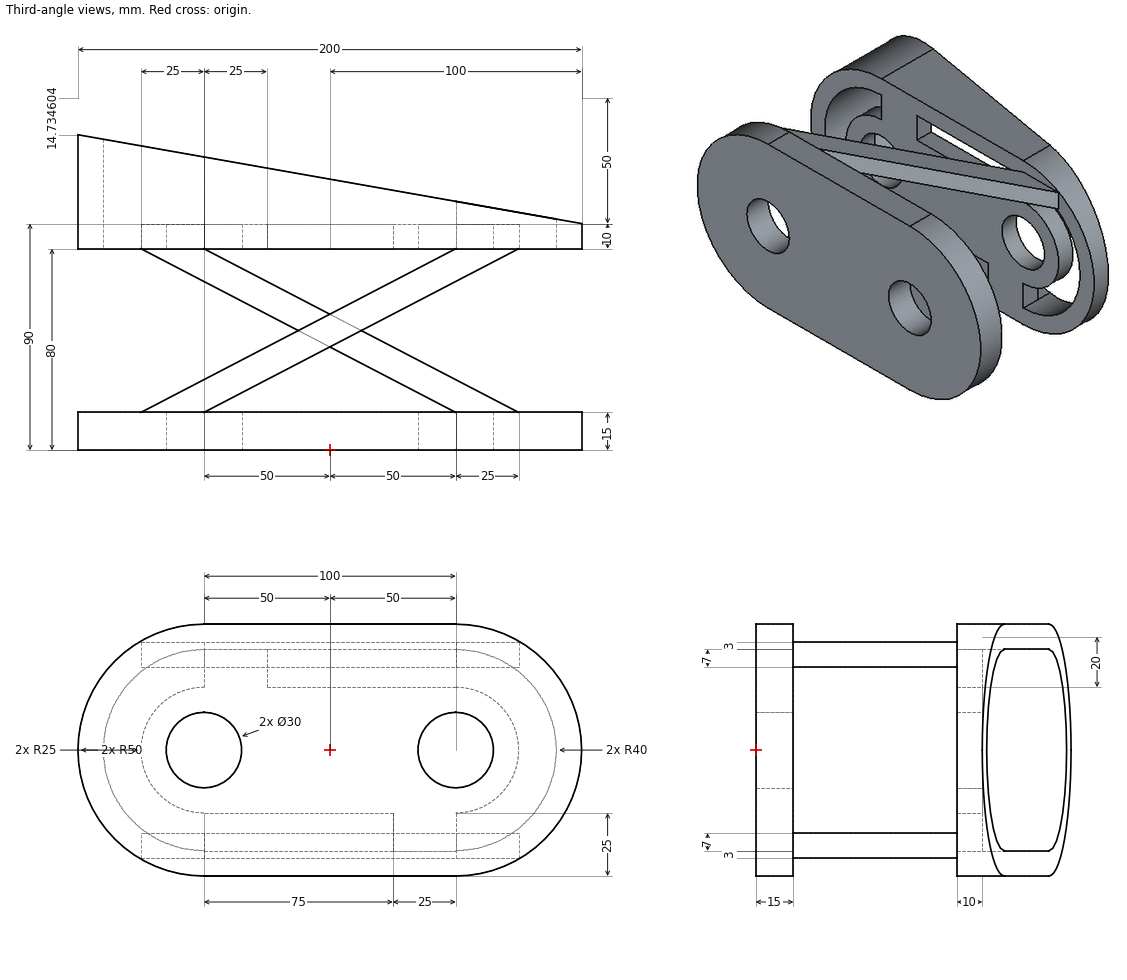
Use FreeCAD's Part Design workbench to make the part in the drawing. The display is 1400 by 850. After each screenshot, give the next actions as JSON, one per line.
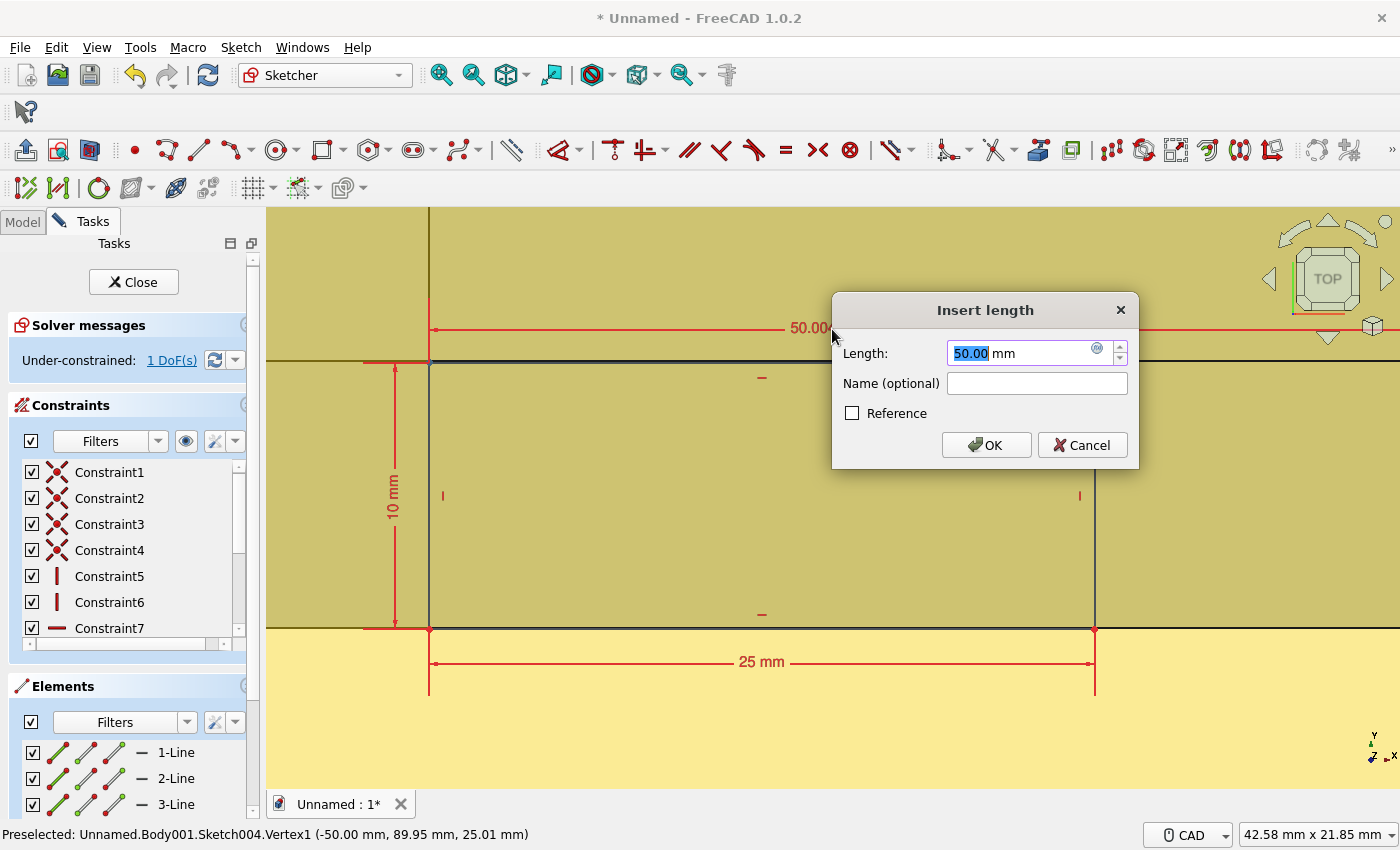
{"action": "type", "text": "50"}
{"action": "key", "text": "Return"}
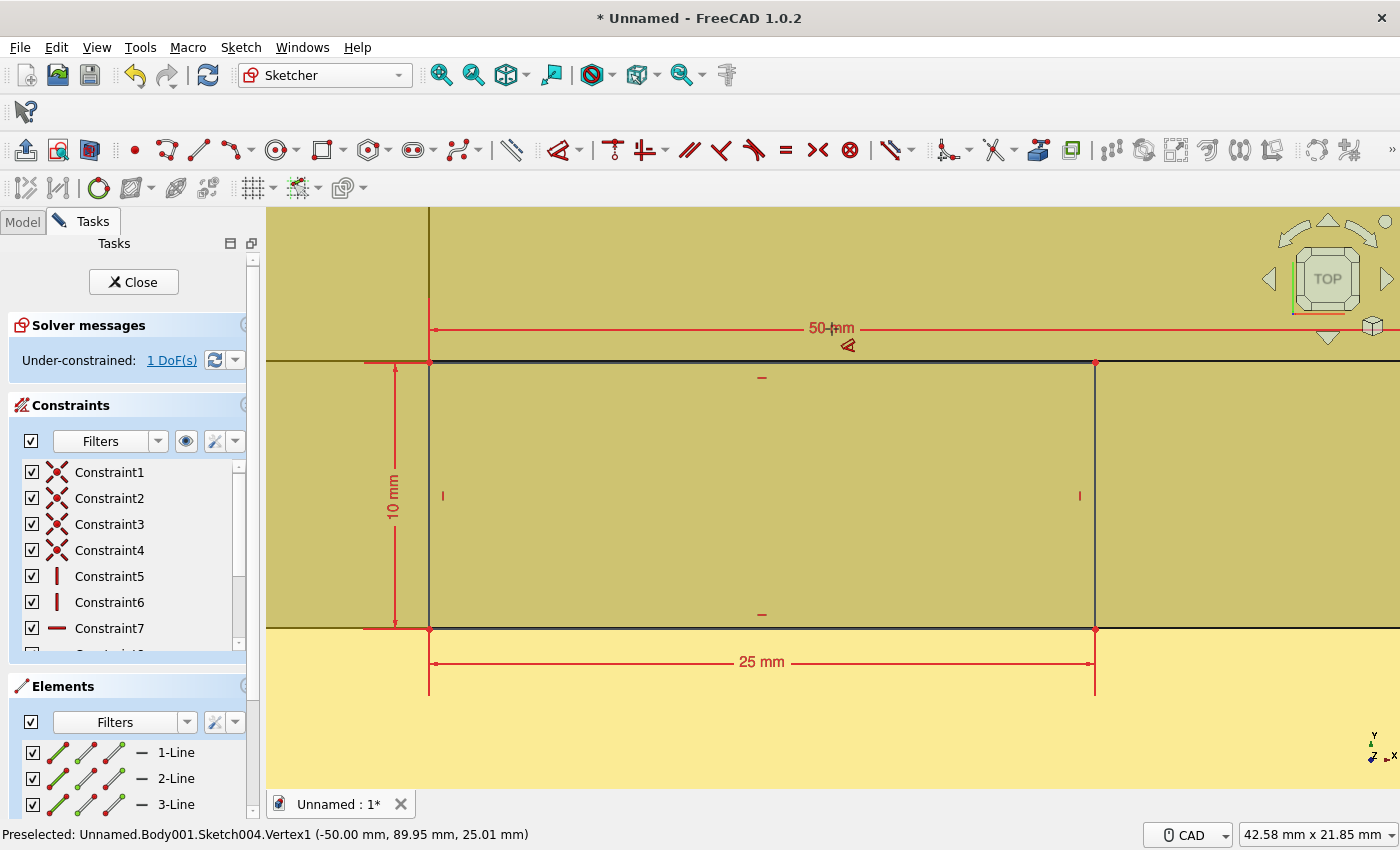
{"action": "left_click", "coordinate": [429, 363]}
{"action": "left_click", "coordinate": [395, 562]}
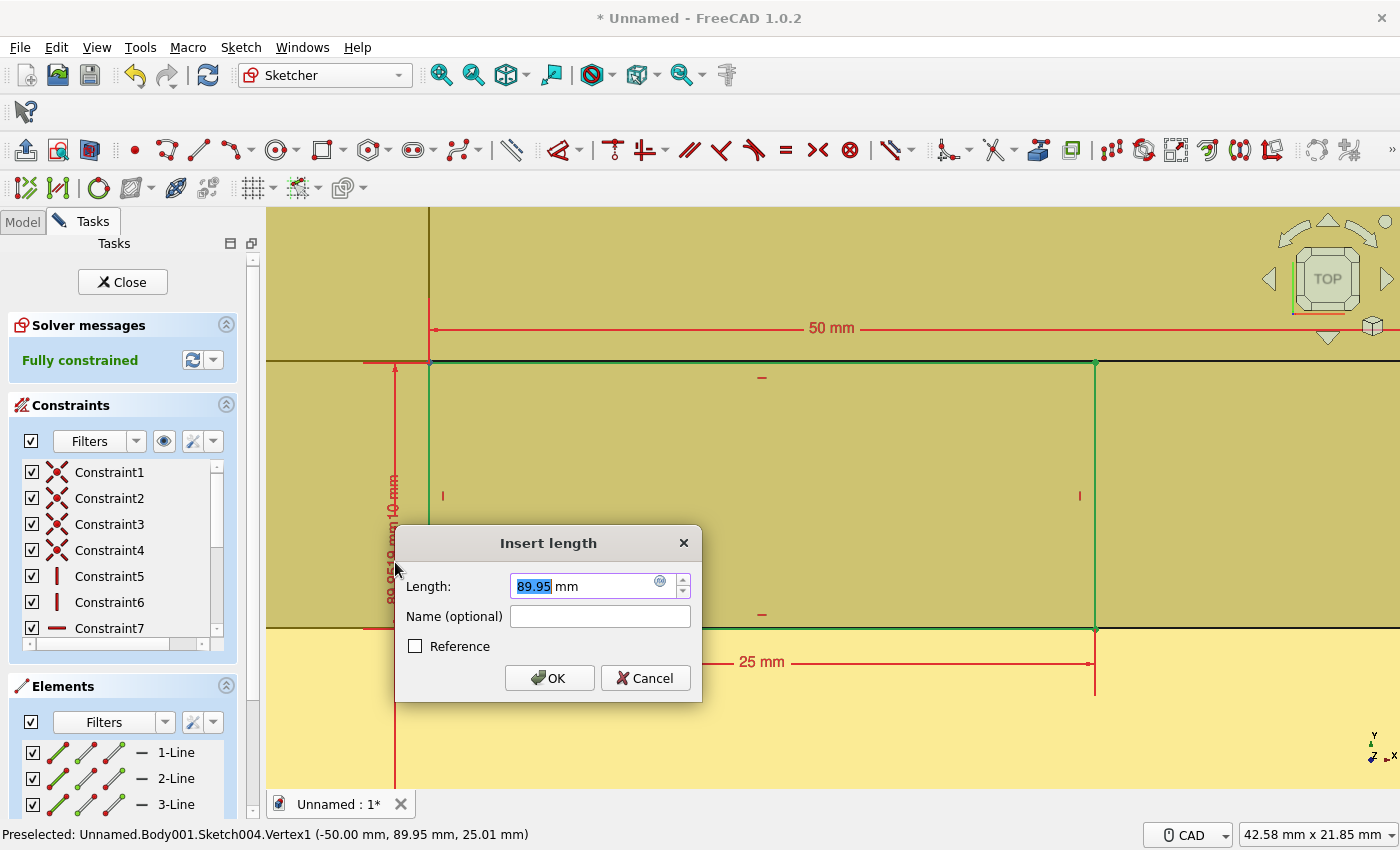
{"action": "type", "text": "90"}
{"action": "key", "text": "Return"}
{"action": "key", "text": "Escape"}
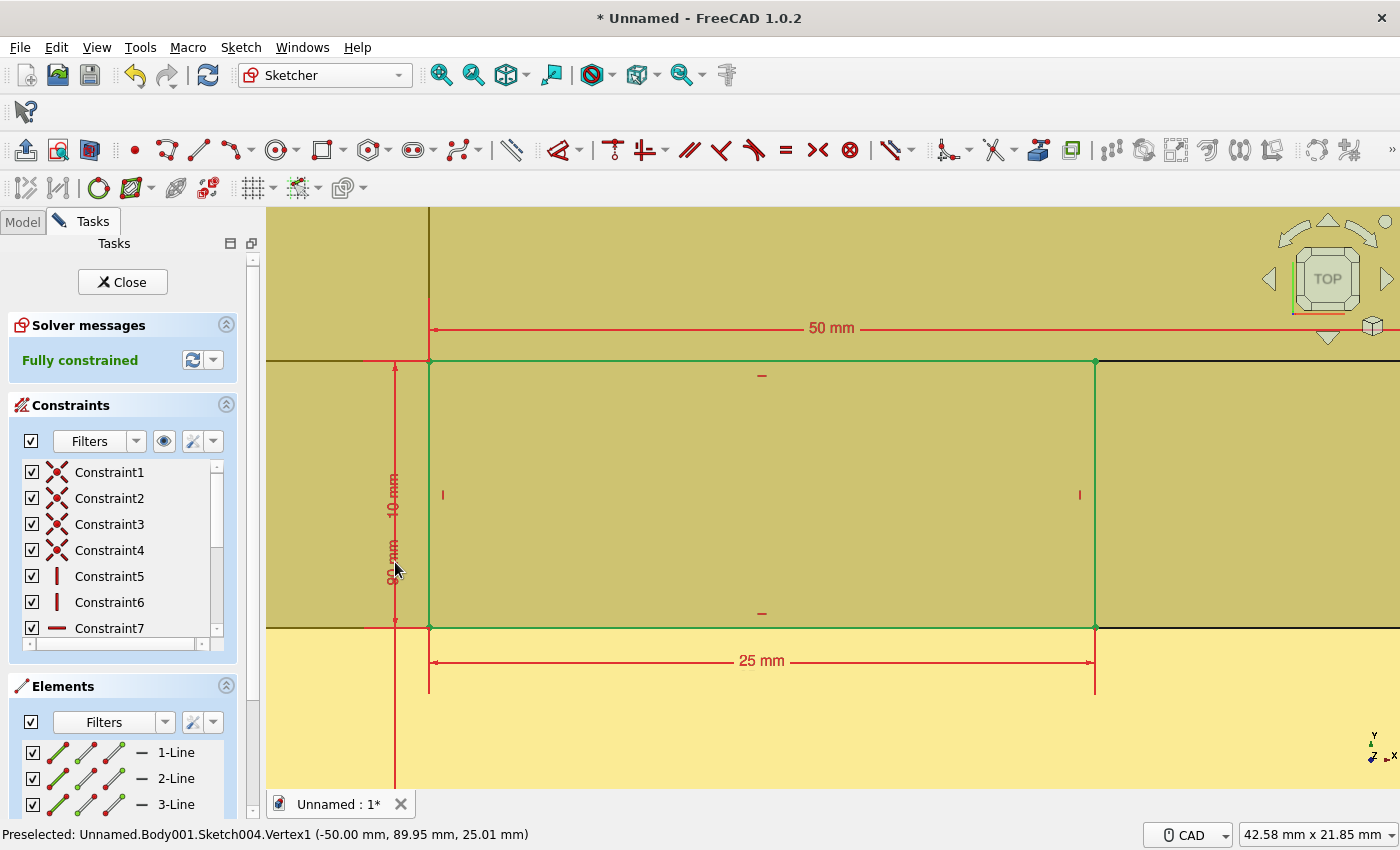
{"action": "left_click", "coordinate": [123, 282]}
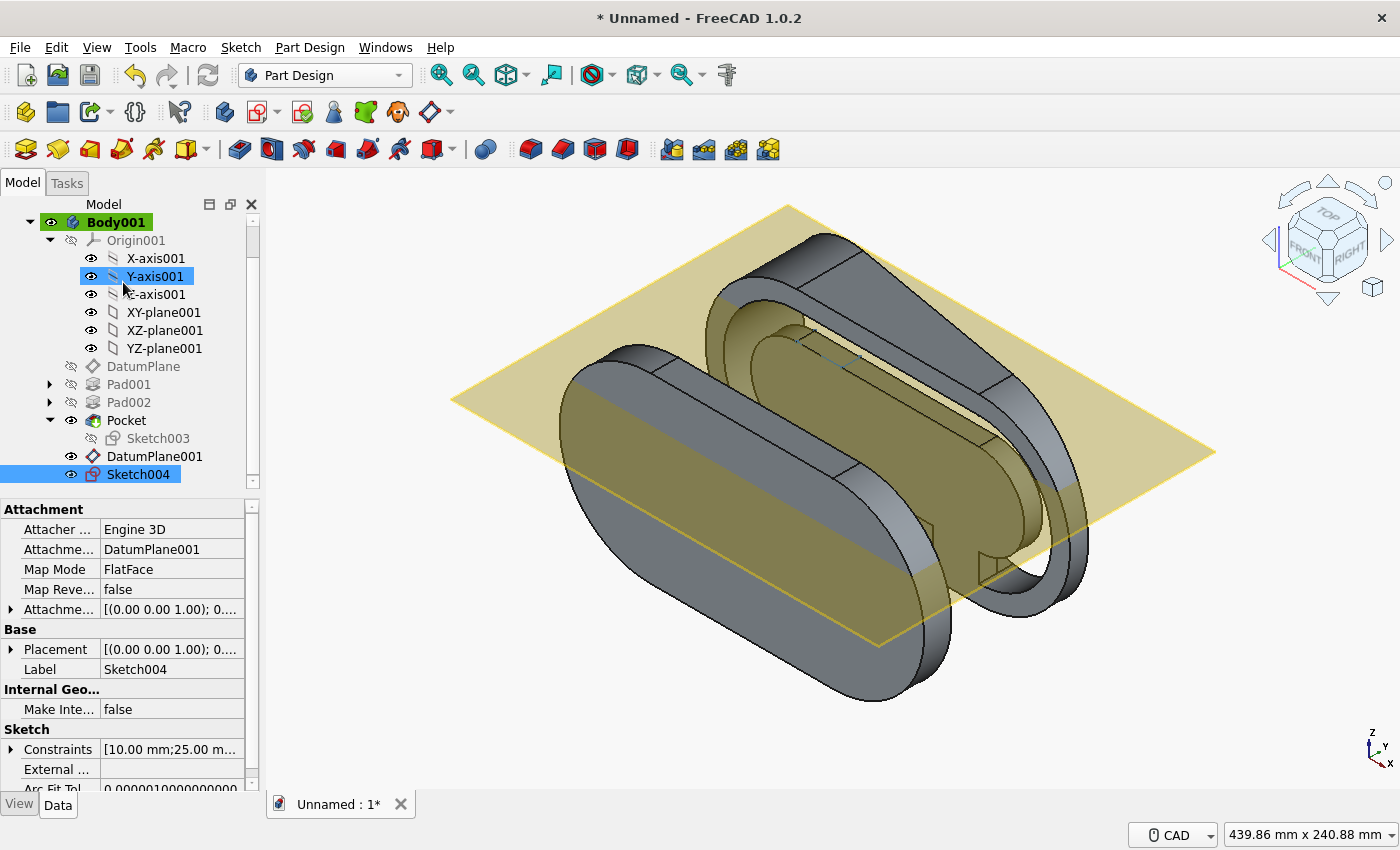
{"action": "left_click", "coordinate": [26, 150]}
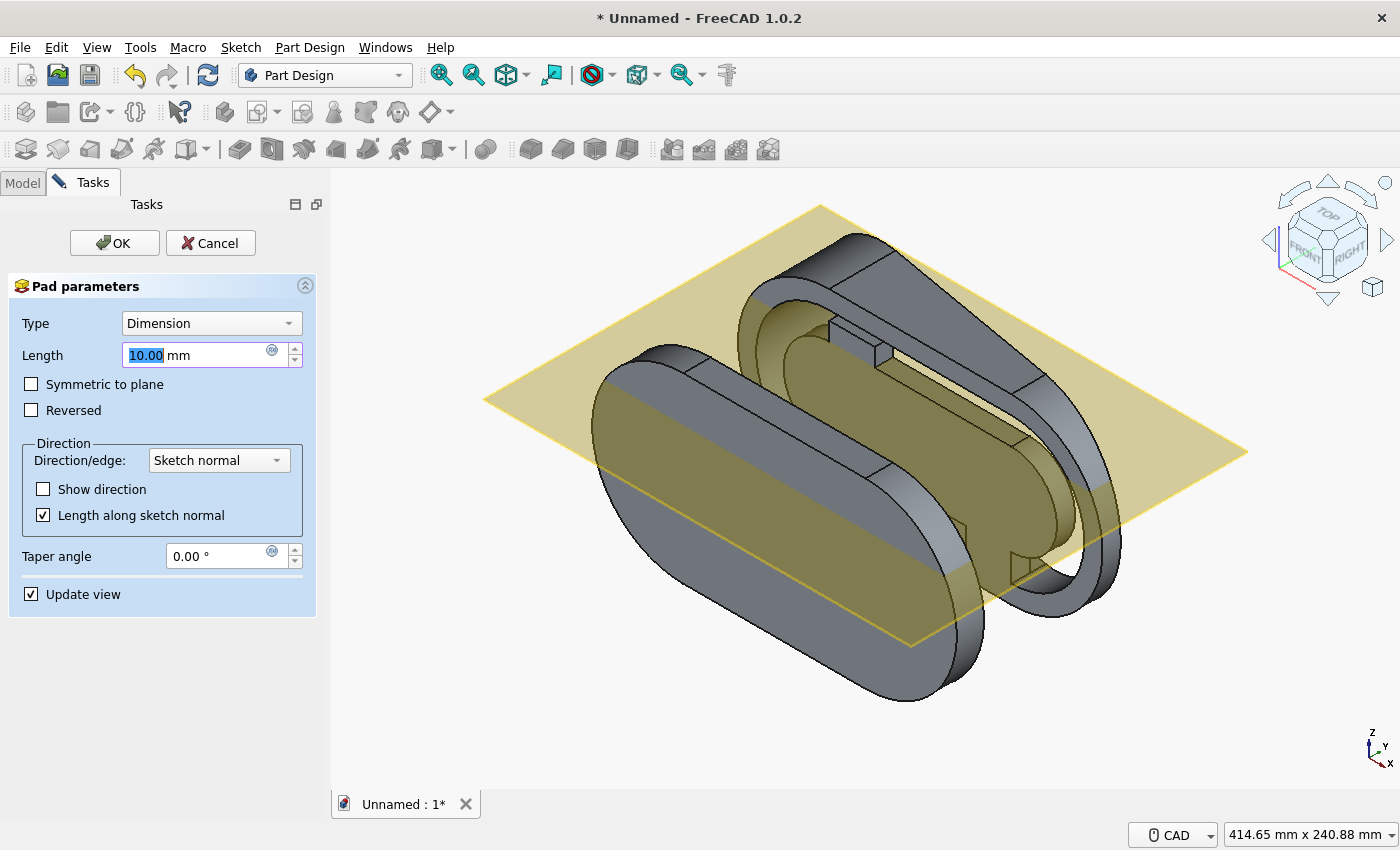
{"action": "type", "text": "20"}
{"action": "key", "text": "Tab"}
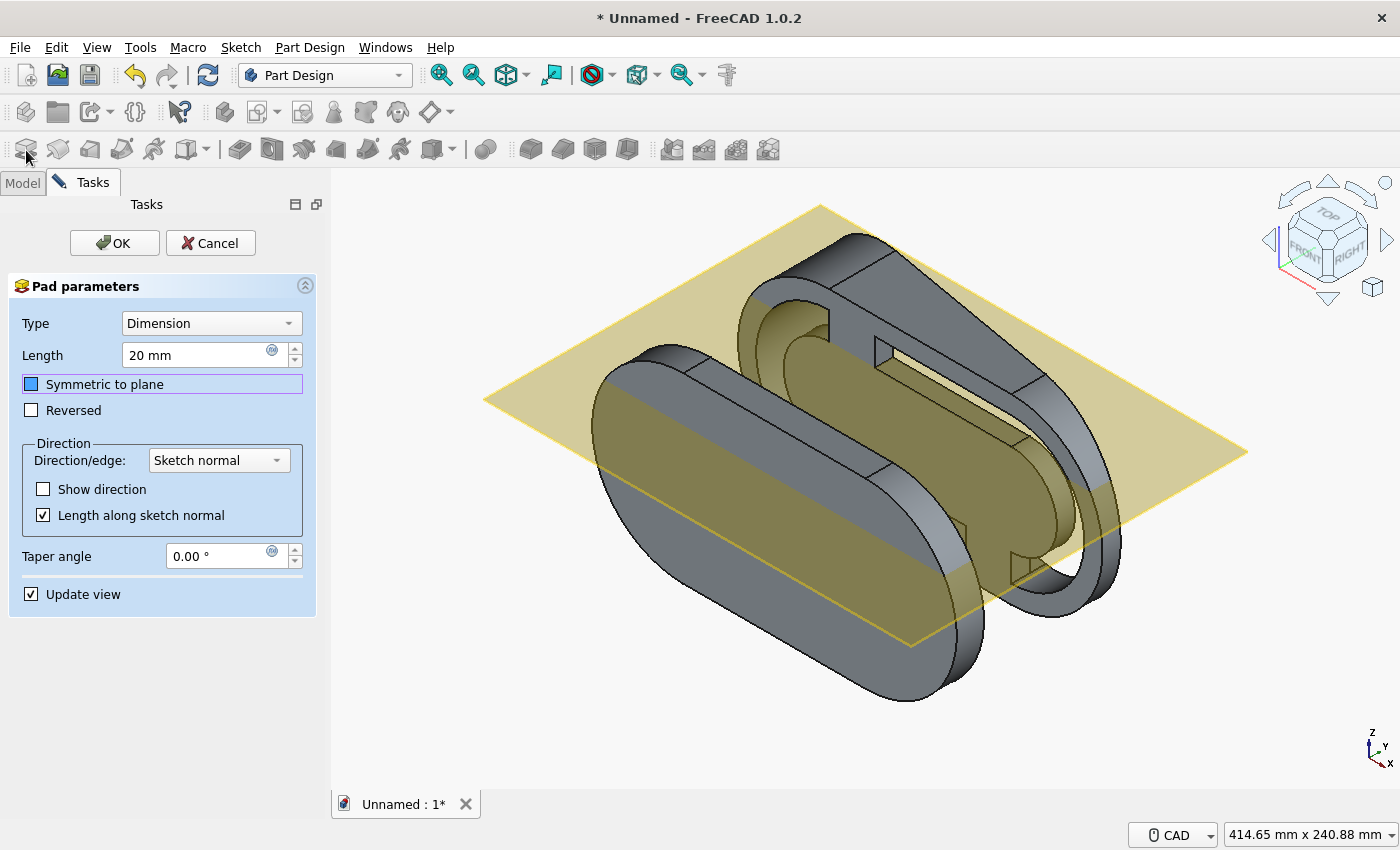
{"action": "left_click", "coordinate": [115, 243]}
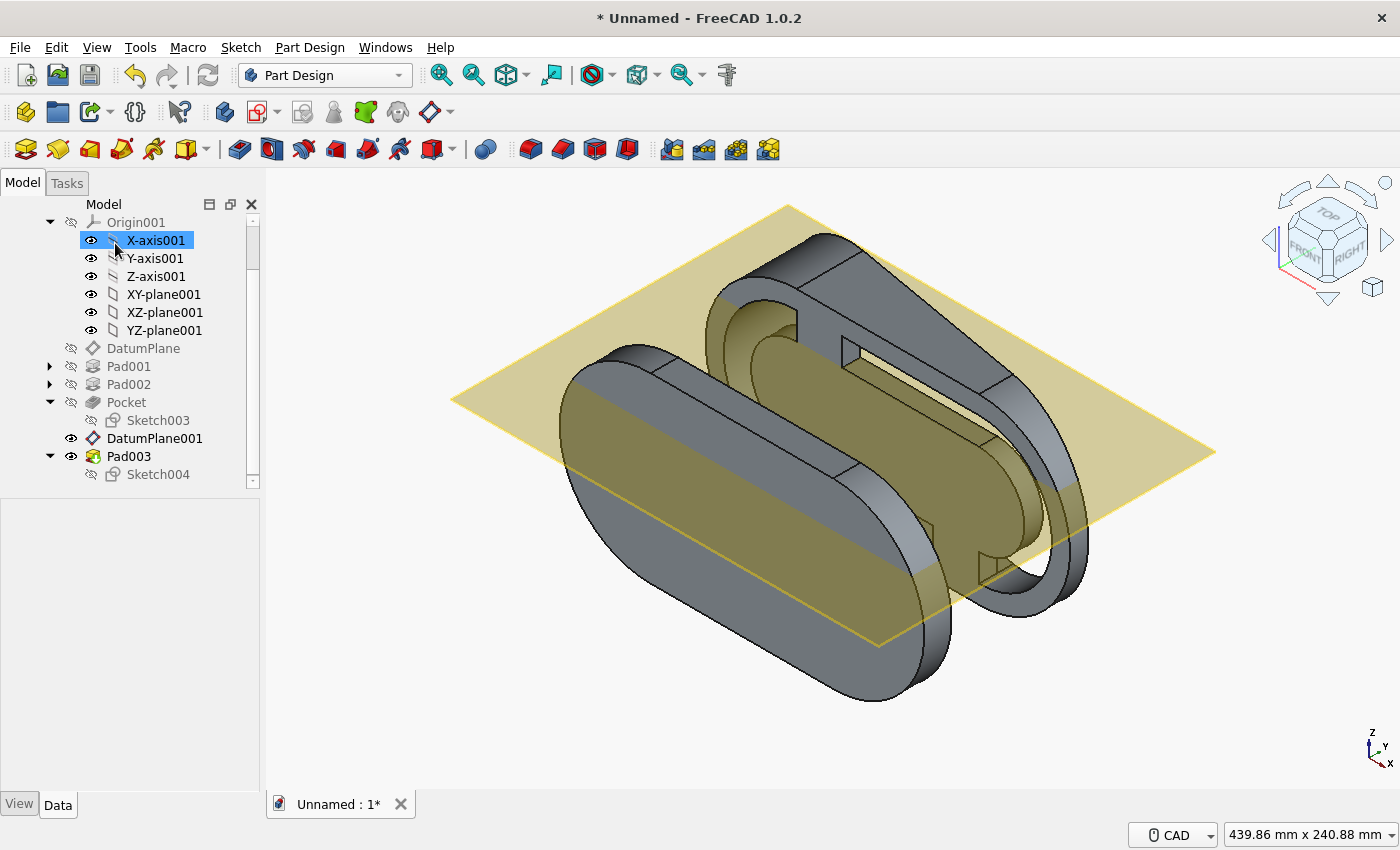
{"action": "left_click", "coordinate": [116, 438]}
{"action": "key", "text": "space"}